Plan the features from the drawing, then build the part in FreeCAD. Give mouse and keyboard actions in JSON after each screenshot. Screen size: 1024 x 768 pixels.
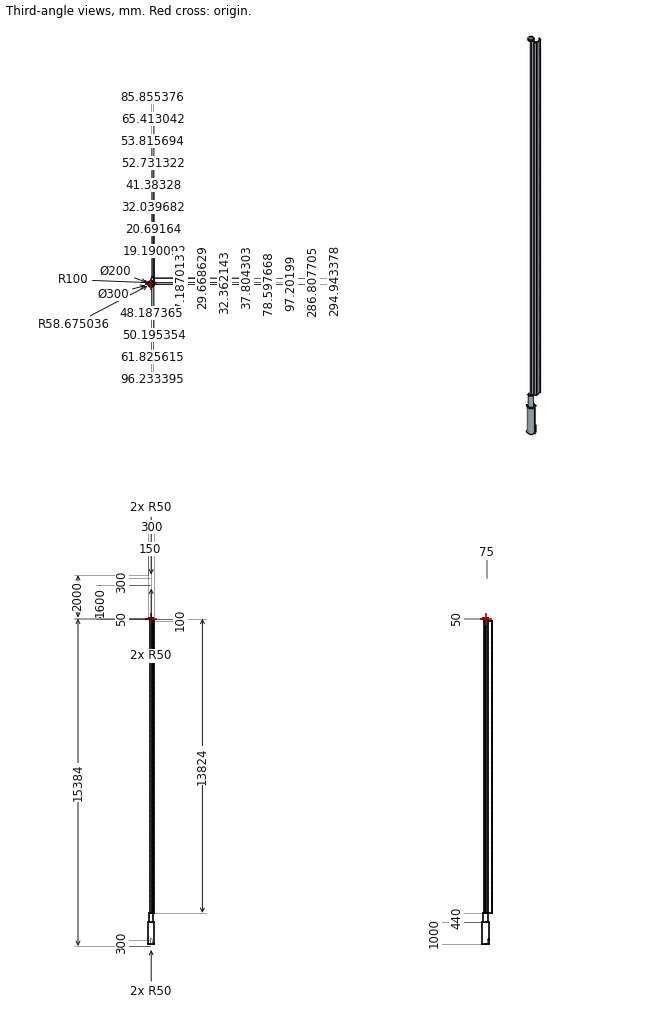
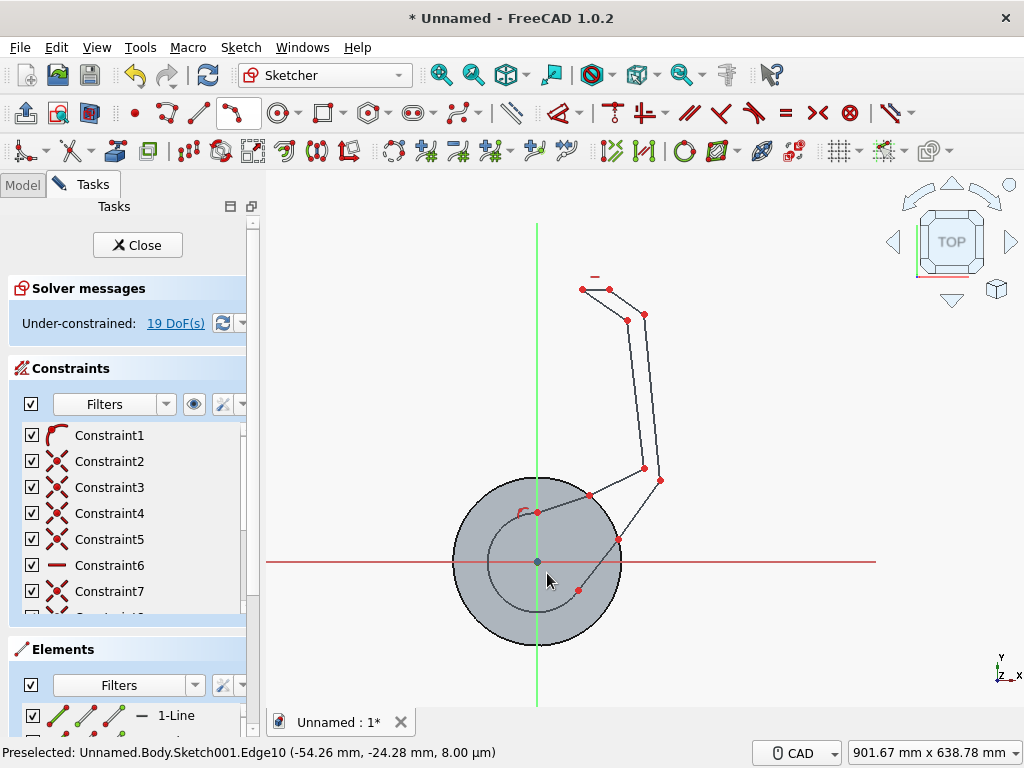
{"action": "left_click", "coordinate": [614, 114]}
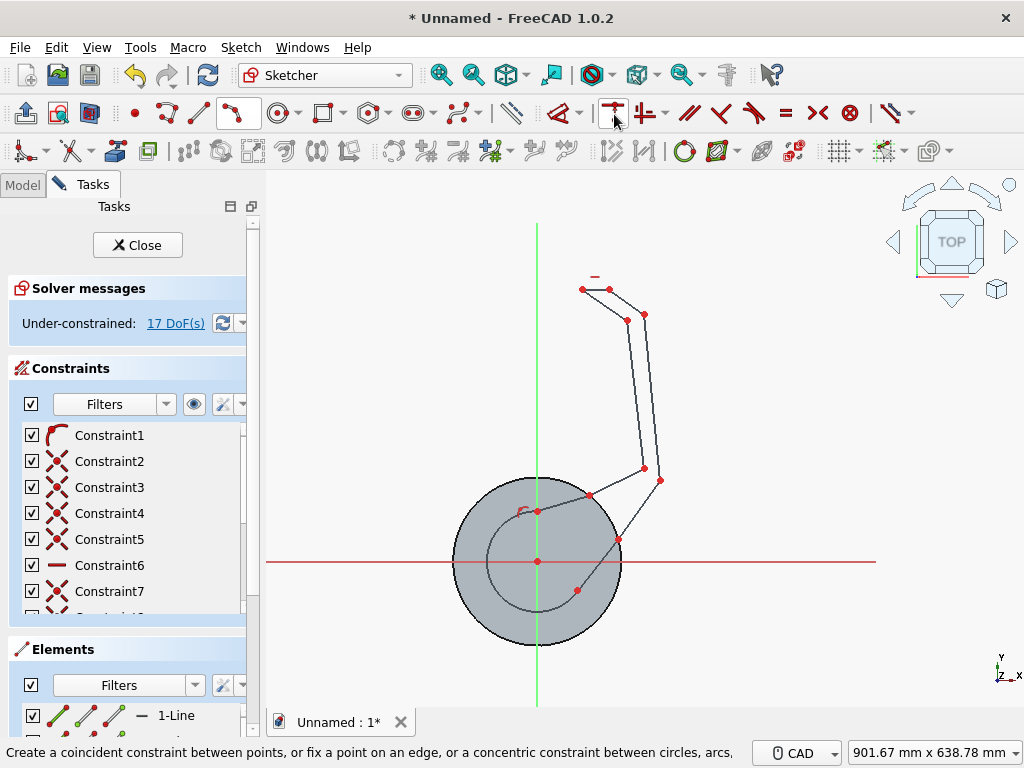
{"action": "left_click", "coordinate": [558, 114]}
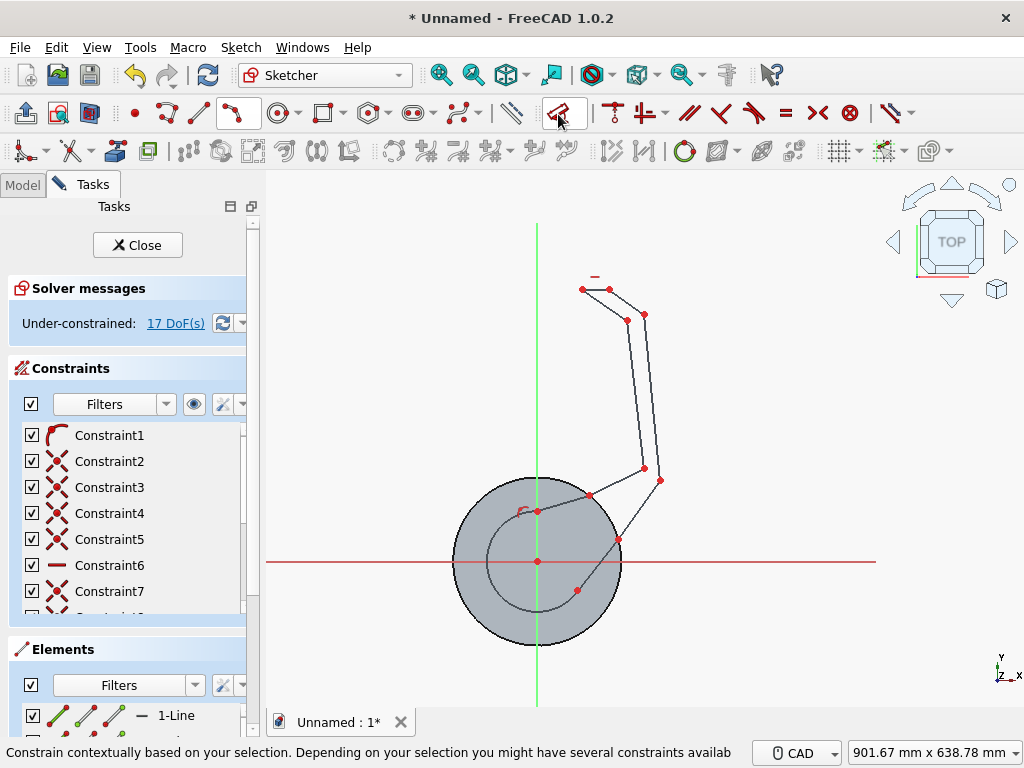
{"action": "left_click", "coordinate": [490, 545]}
{"action": "left_click", "coordinate": [460, 534]}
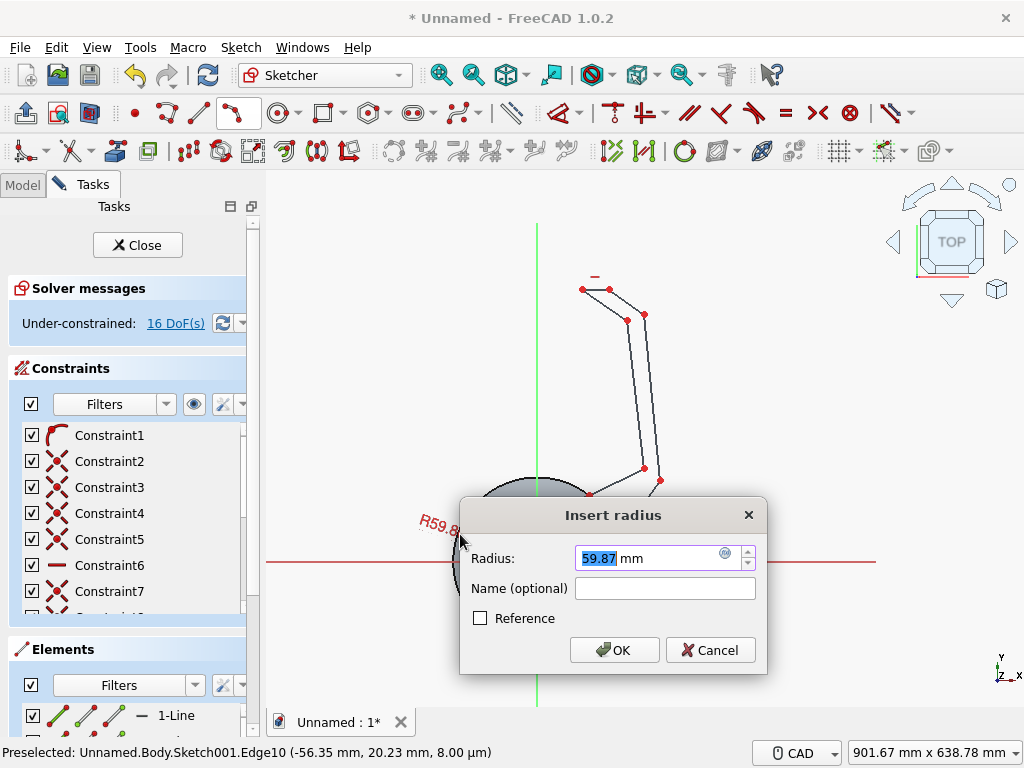
{"action": "type", "text": "58.675036"}
{"action": "key", "text": "Return"}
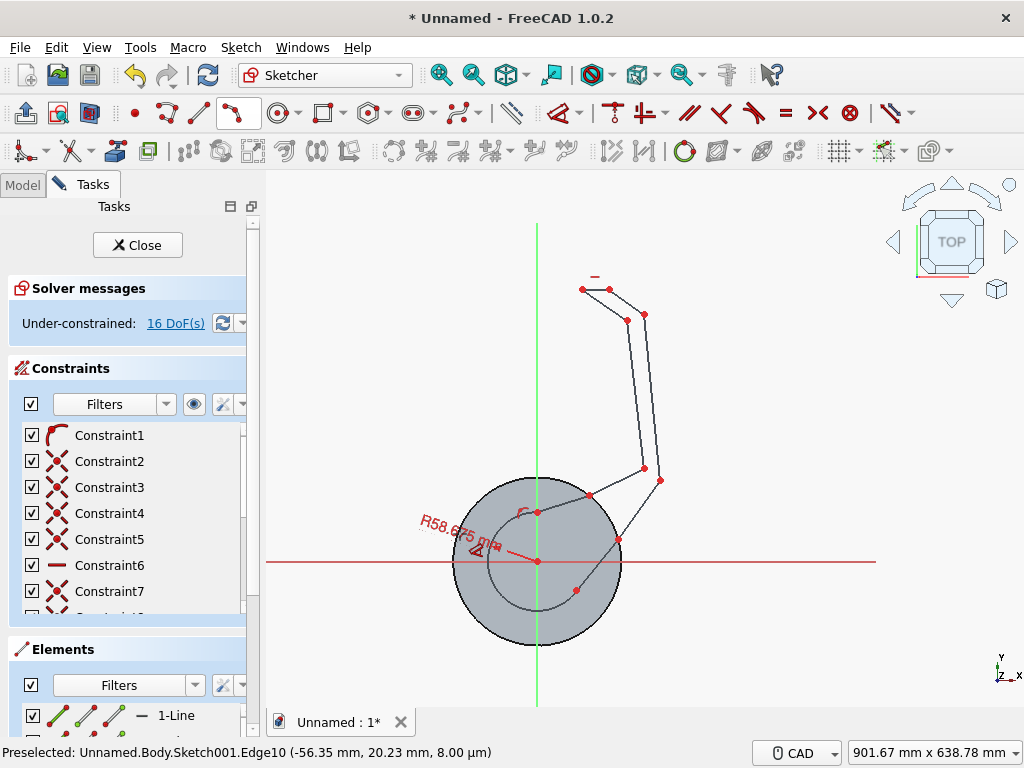
{"action": "scroll", "coordinate": [598, 290], "scroll_direction": "up", "scroll_amount": 3}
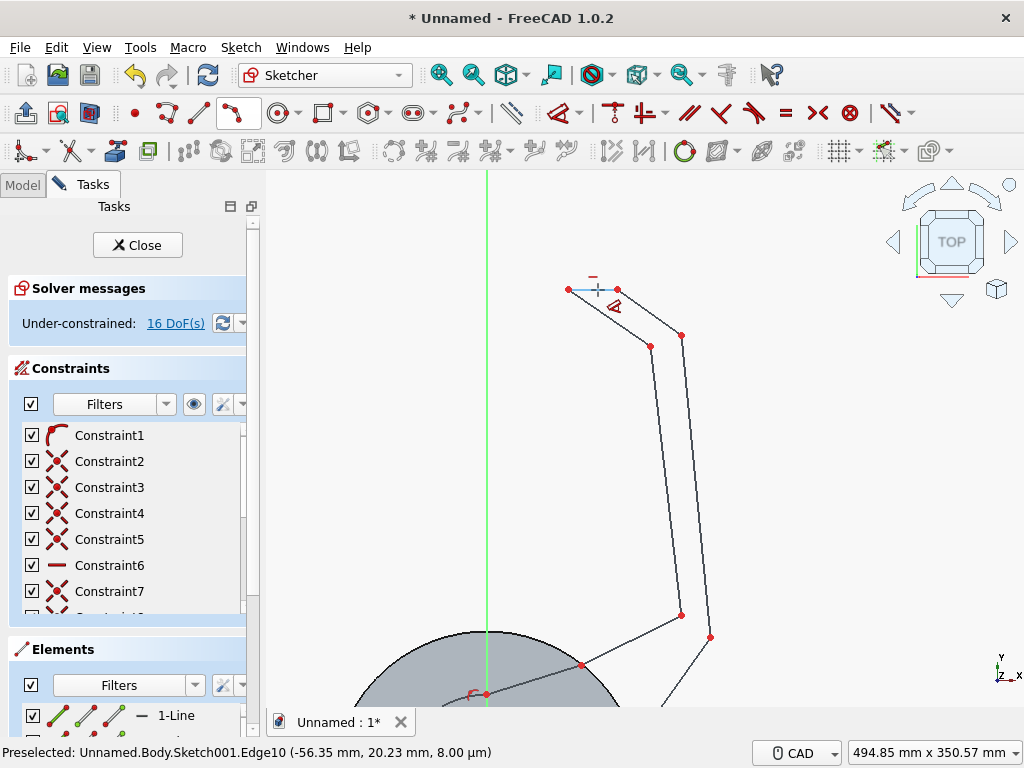
{"action": "left_click", "coordinate": [598, 290]}
{"action": "left_click", "coordinate": [593, 256]}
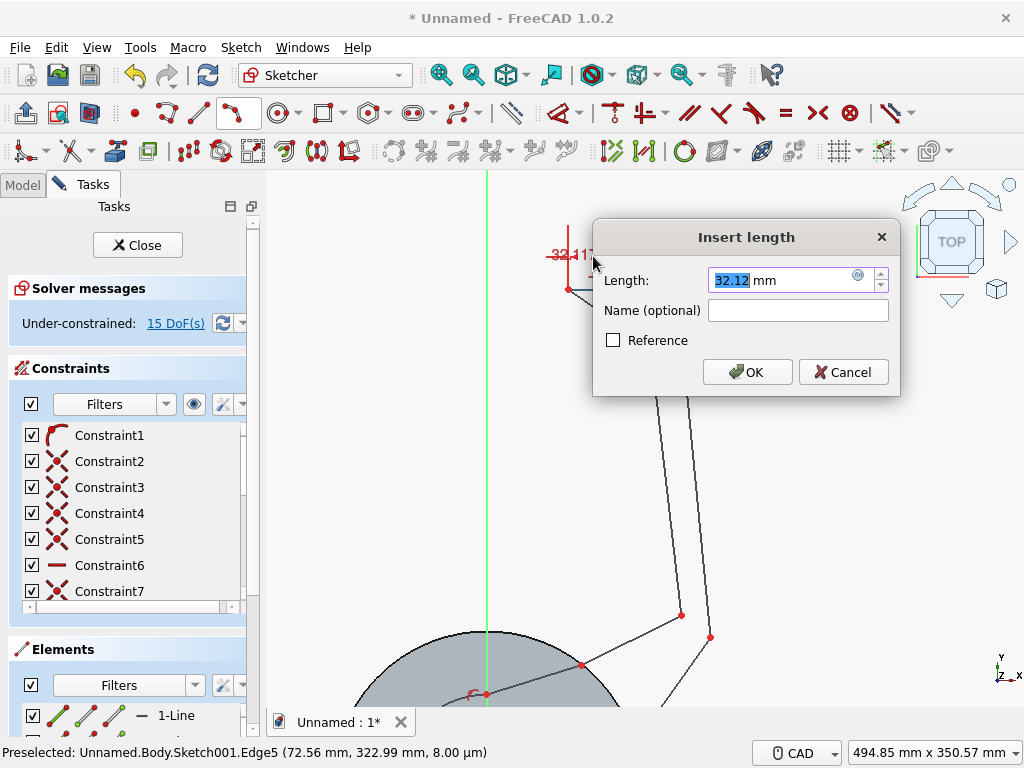
{"action": "type", "text": "32.039682"}
{"action": "key", "text": "Return"}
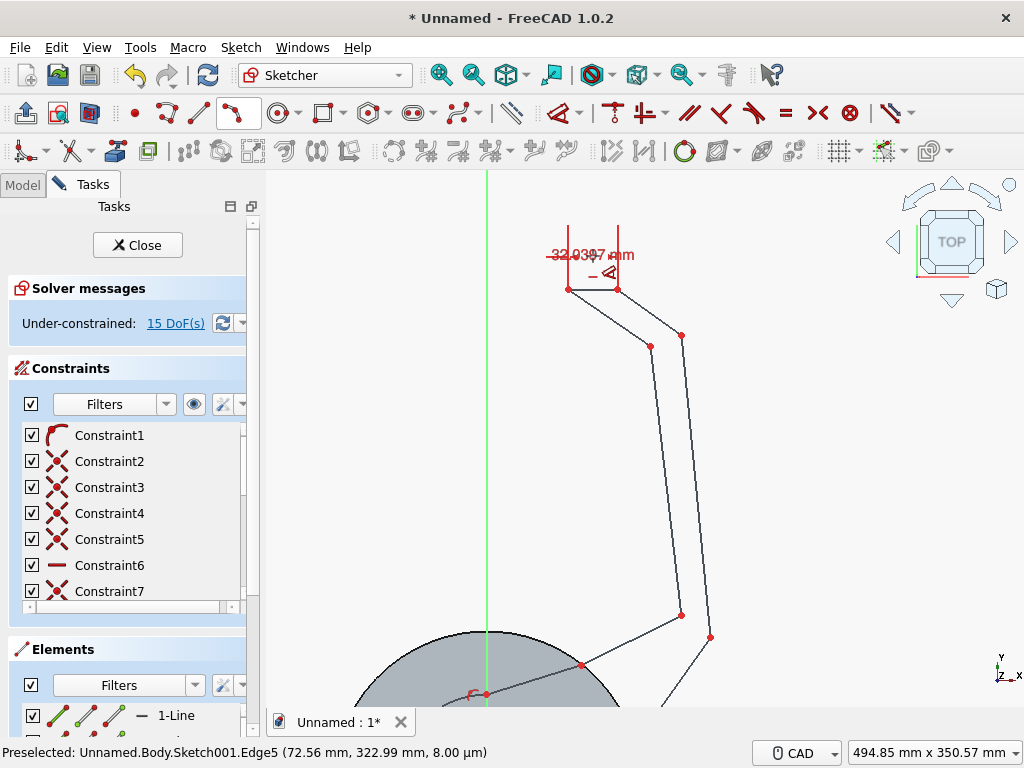
{"action": "left_click", "coordinate": [711, 638]}
{"action": "left_click", "coordinate": [745, 658]}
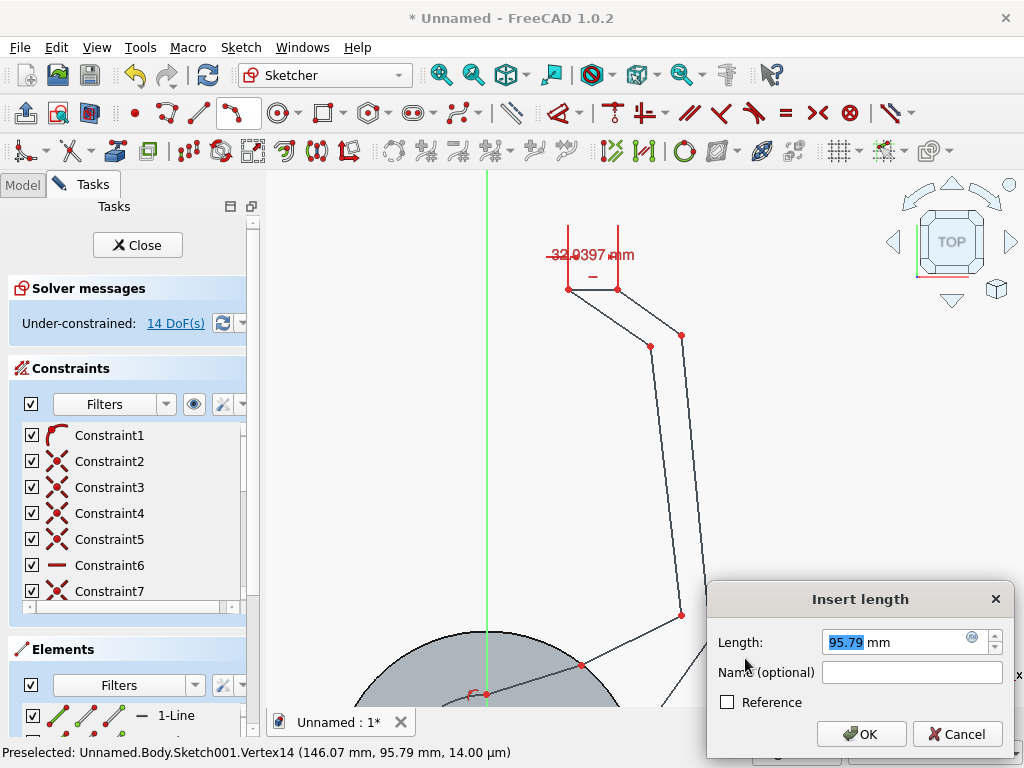
{"action": "type", "text": "97.20199"}
{"action": "key", "text": "Return"}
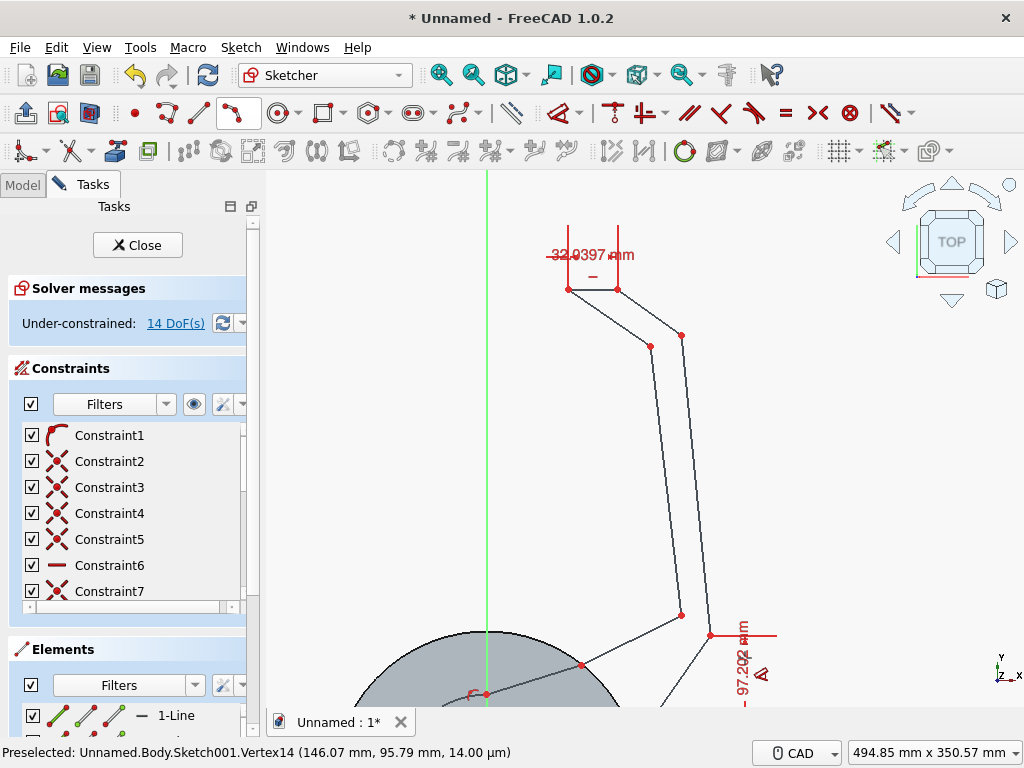
{"action": "scroll", "coordinate": [672, 535], "scroll_direction": "up", "scroll_amount": 2}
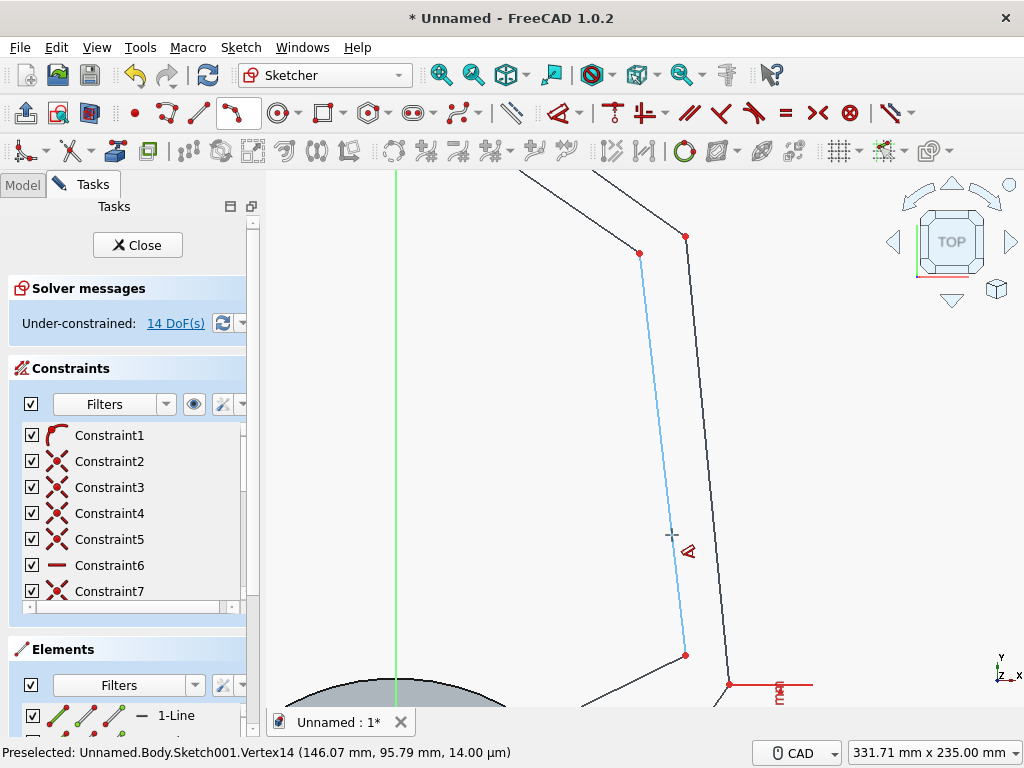
{"action": "left_click", "coordinate": [672, 535]}
{"action": "left_click", "coordinate": [673, 219]}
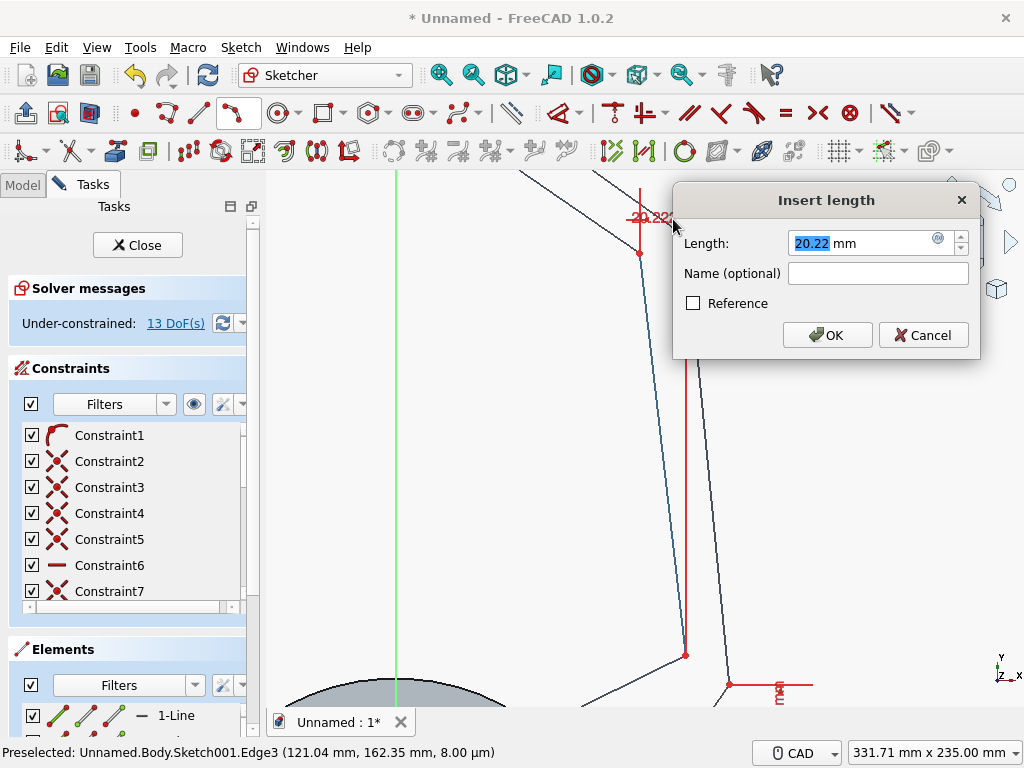
{"action": "type", "text": "20.69164"}
{"action": "key", "text": "Return"}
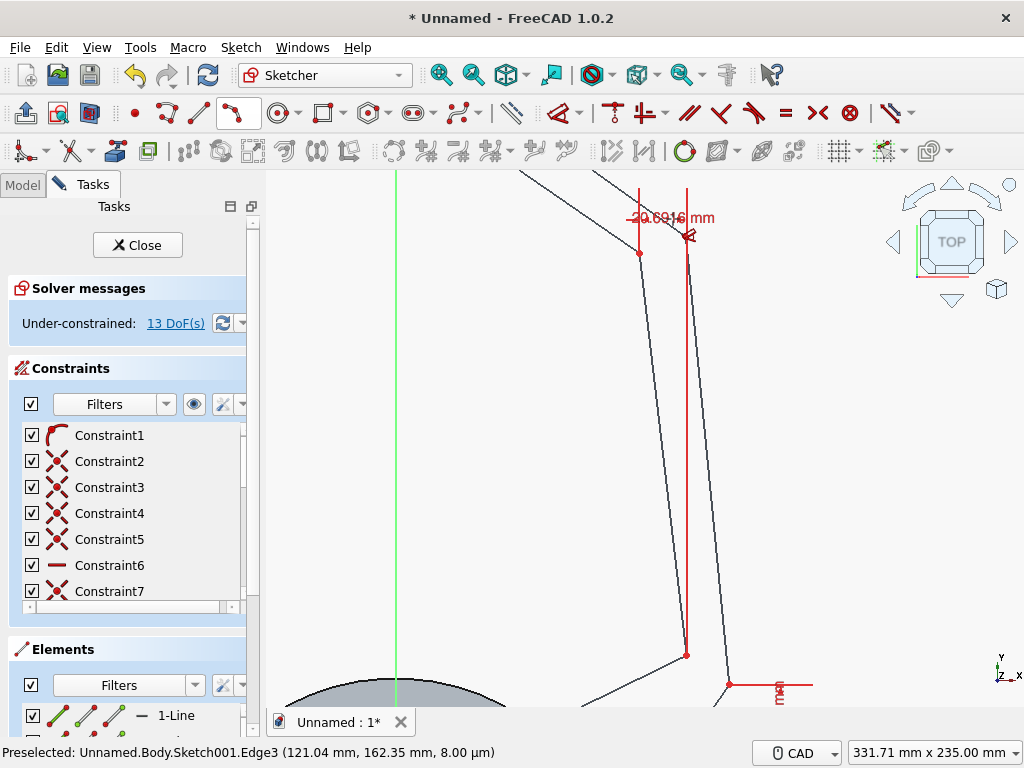
{"action": "left_click", "coordinate": [657, 216]}
{"action": "left_click", "coordinate": [616, 271]}